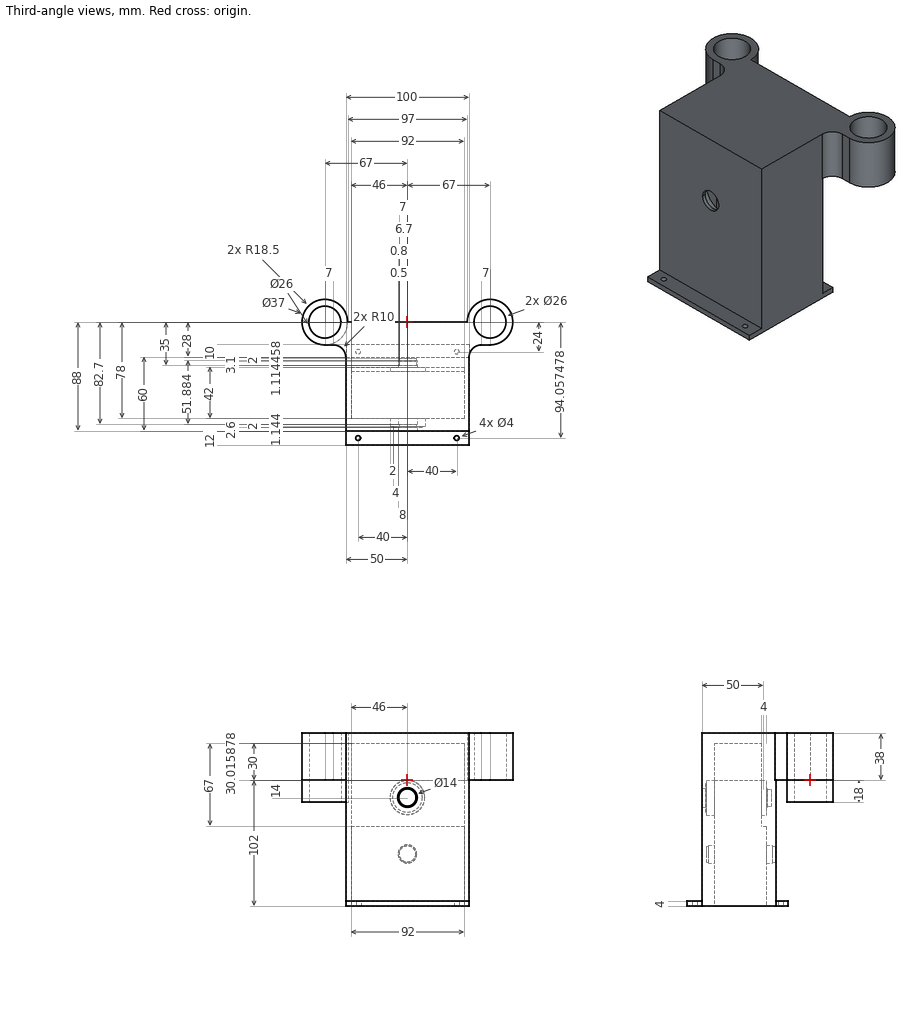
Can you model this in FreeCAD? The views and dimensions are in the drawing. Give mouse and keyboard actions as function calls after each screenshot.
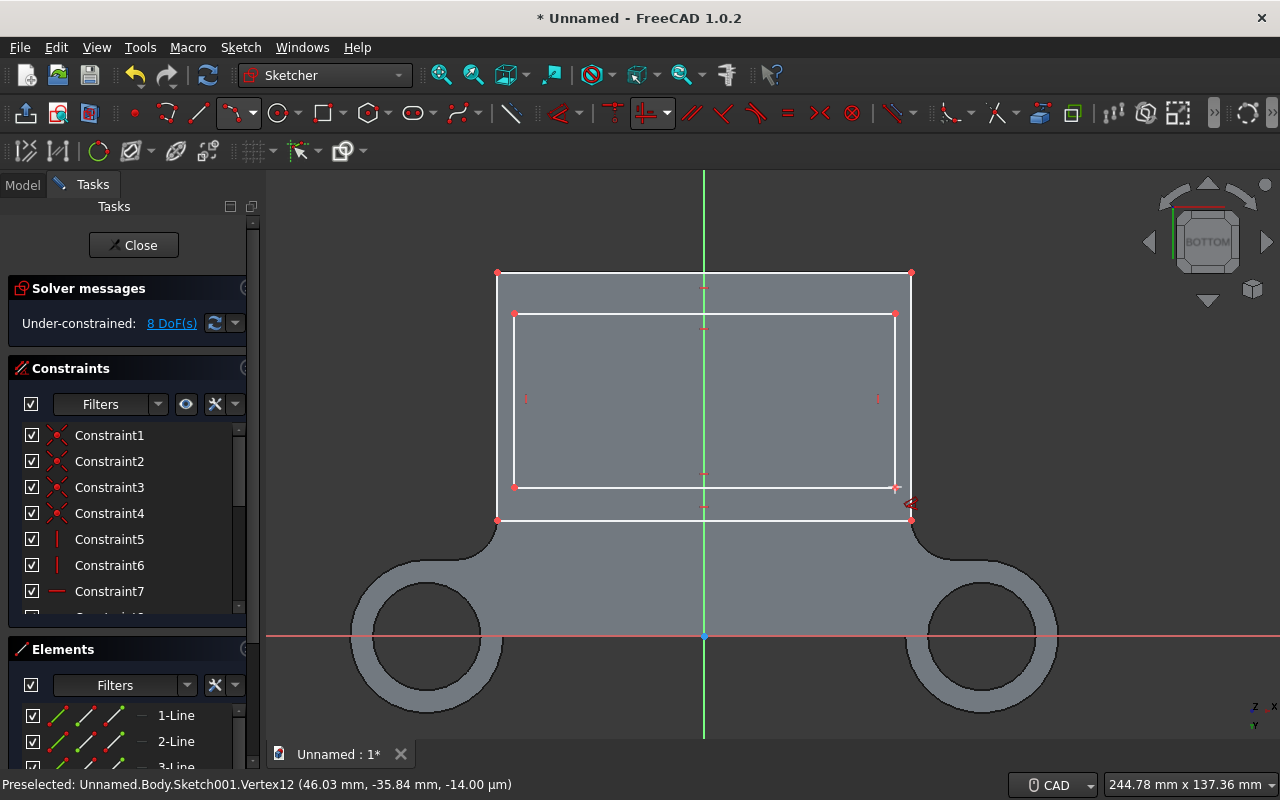
click(497, 347)
click(463, 397)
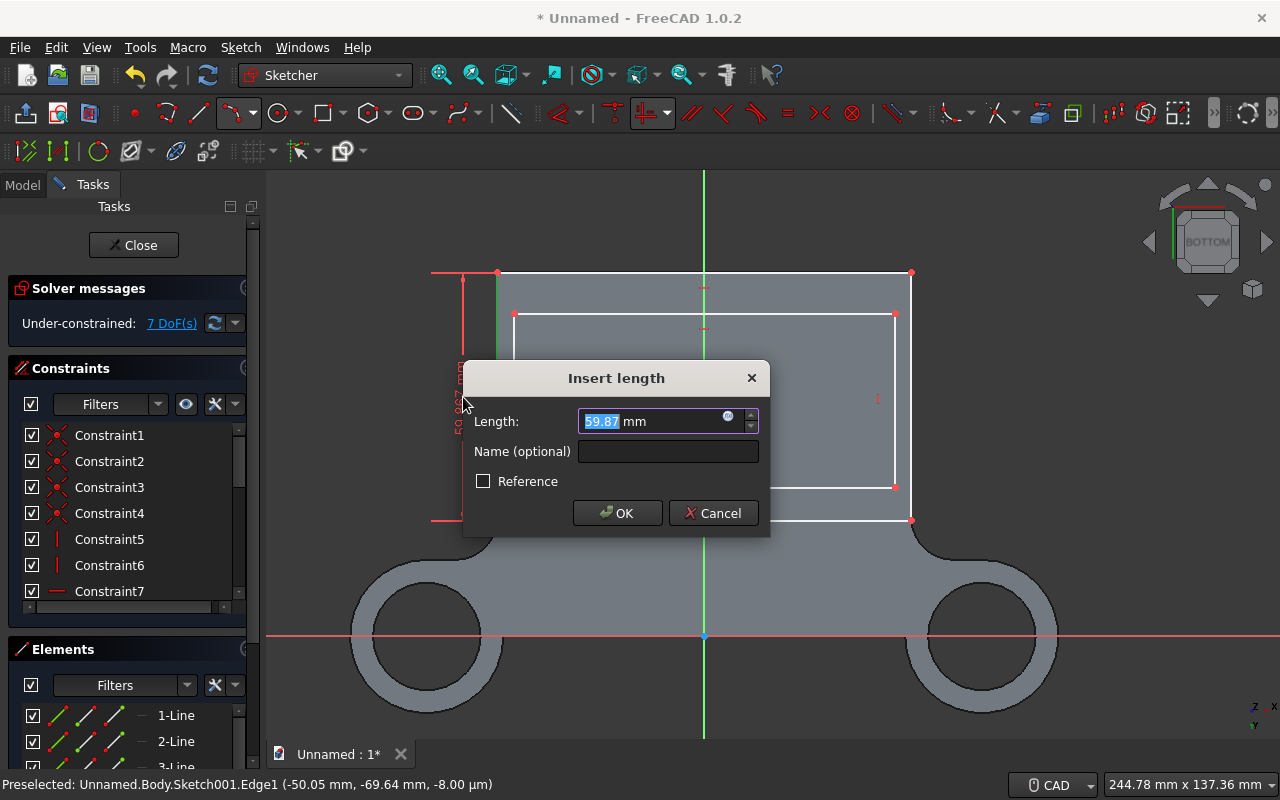
text(60)
key(Return)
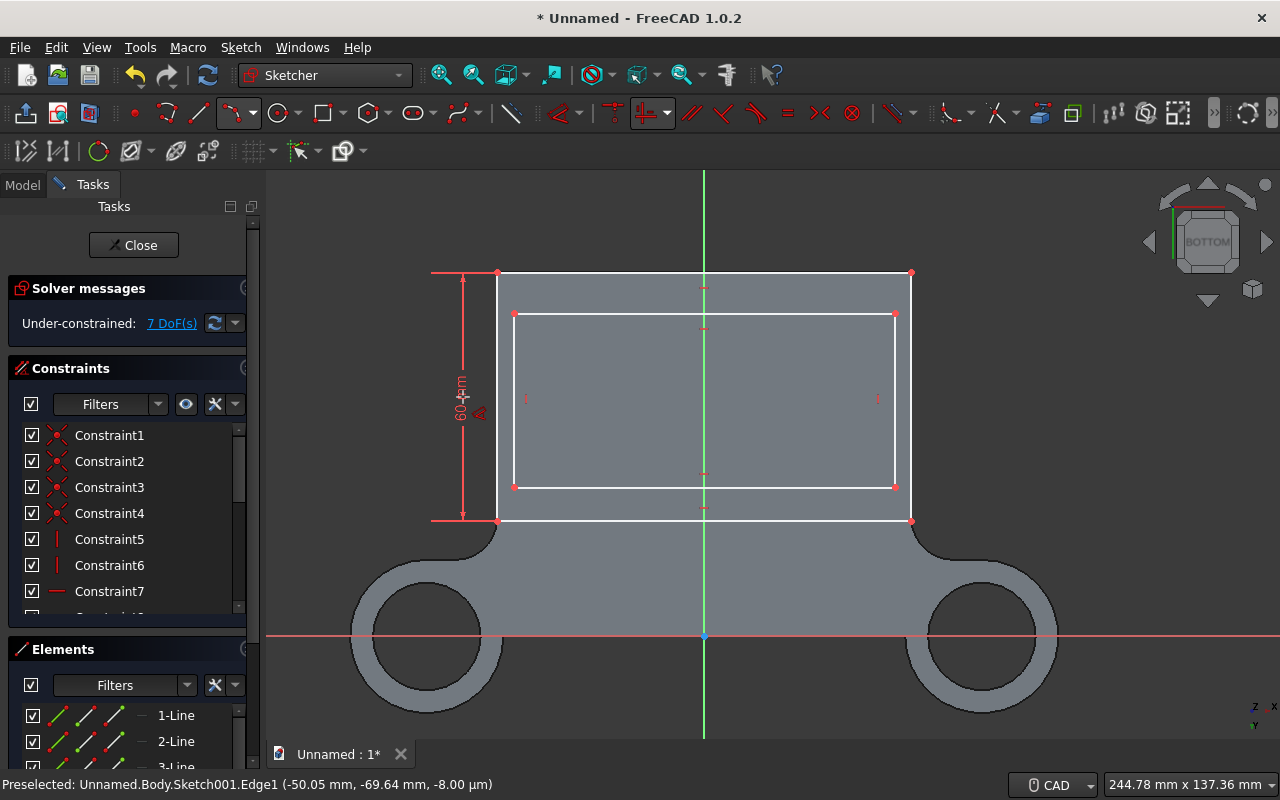
click(514, 366)
click(480, 361)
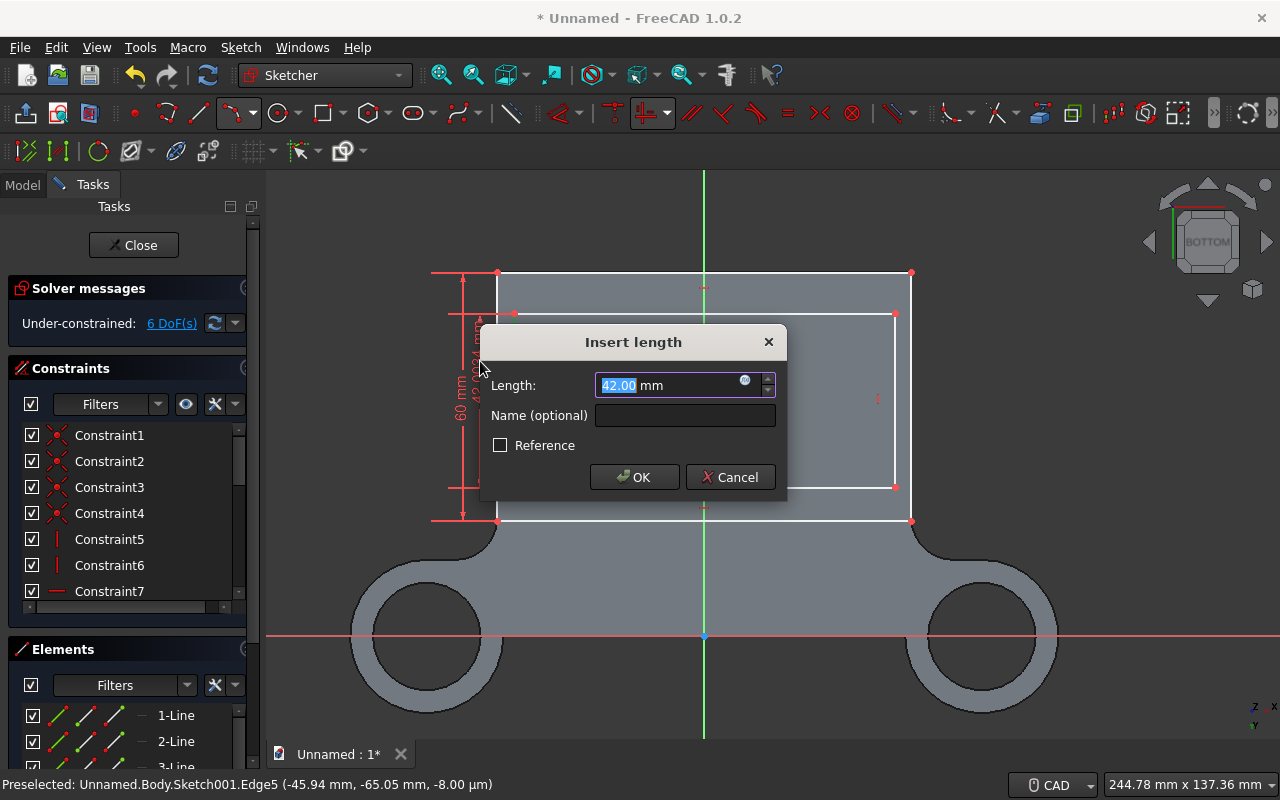
text(42)
key(Return)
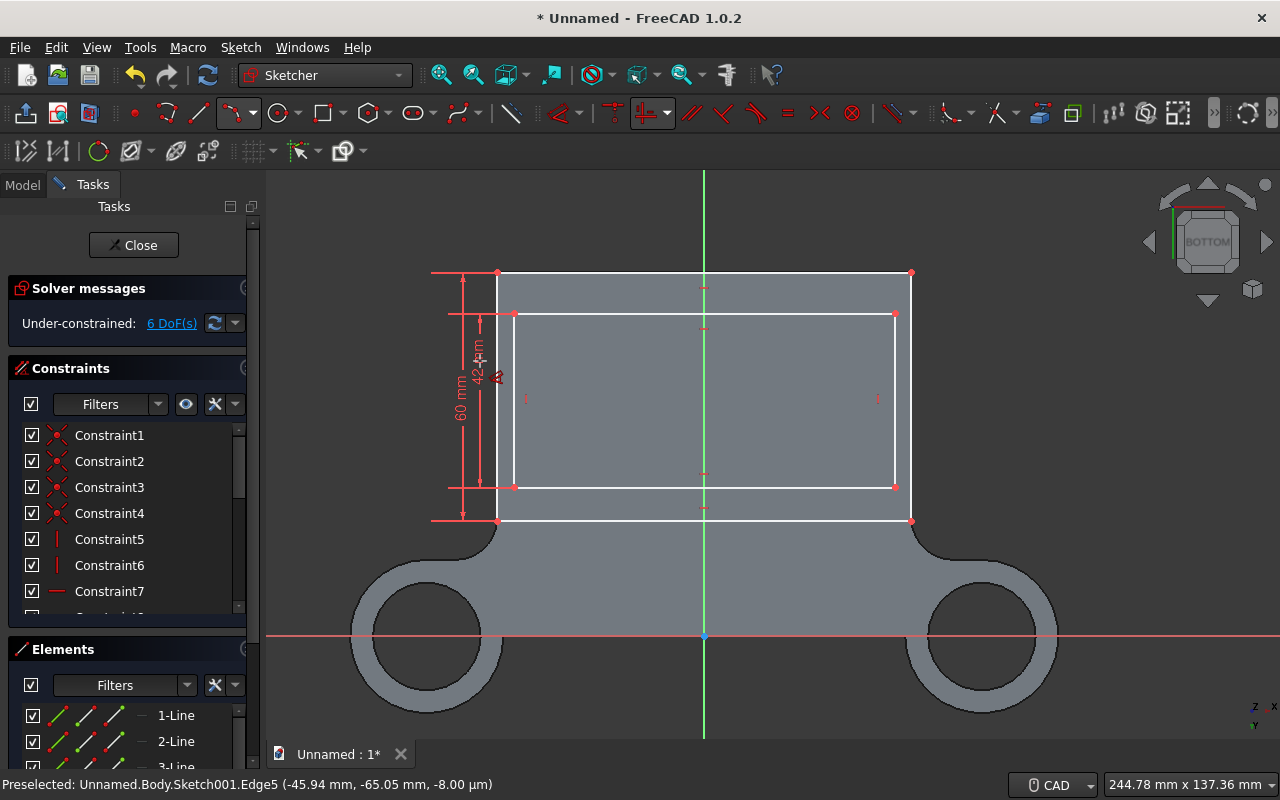
click(628, 488)
click(617, 454)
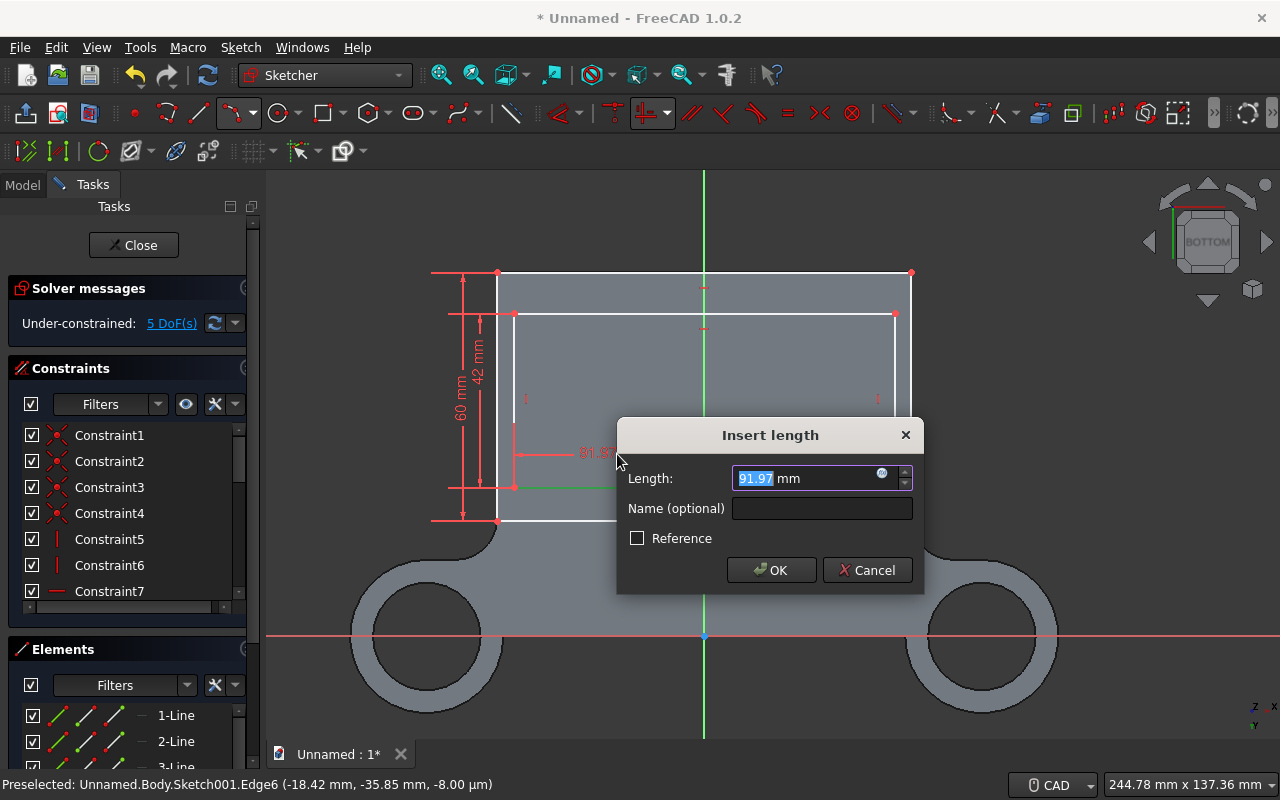
text(92)
key(Return)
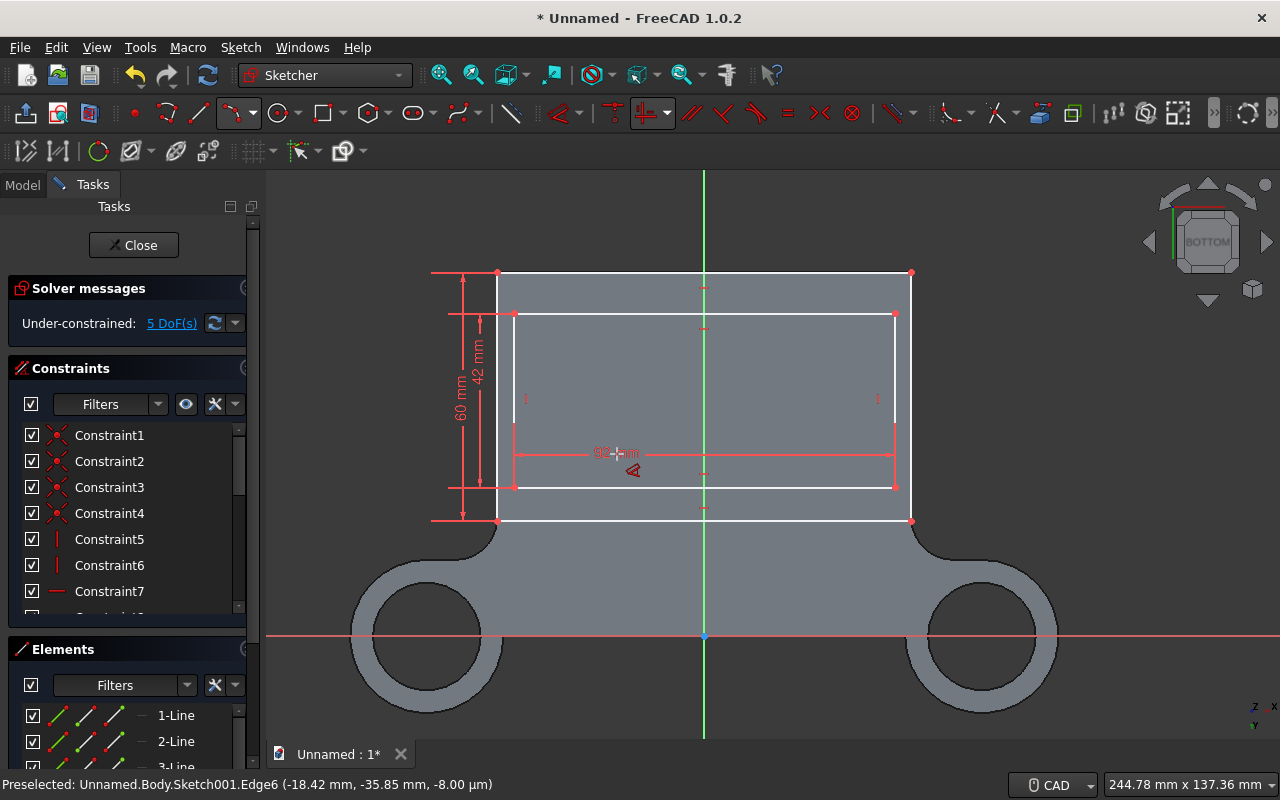
click(621, 521)
click(609, 555)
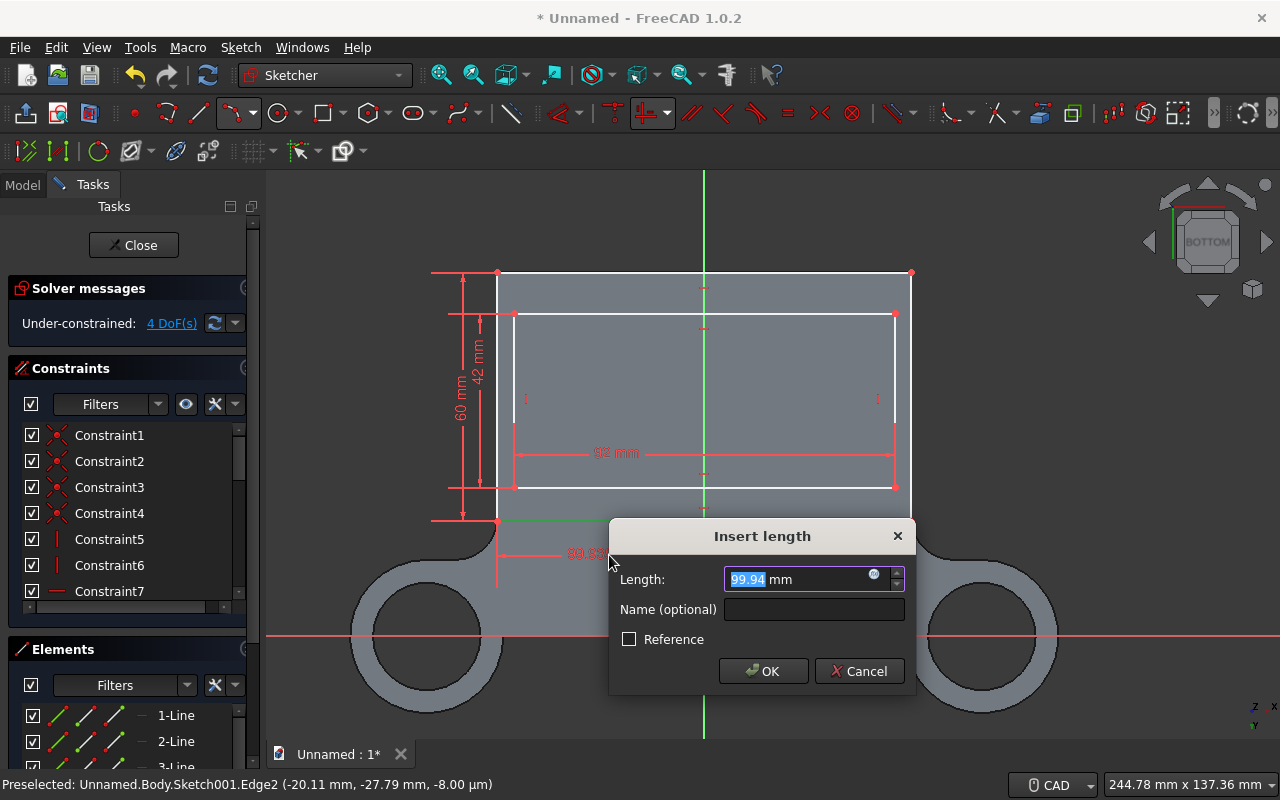
text(100)
key(Return)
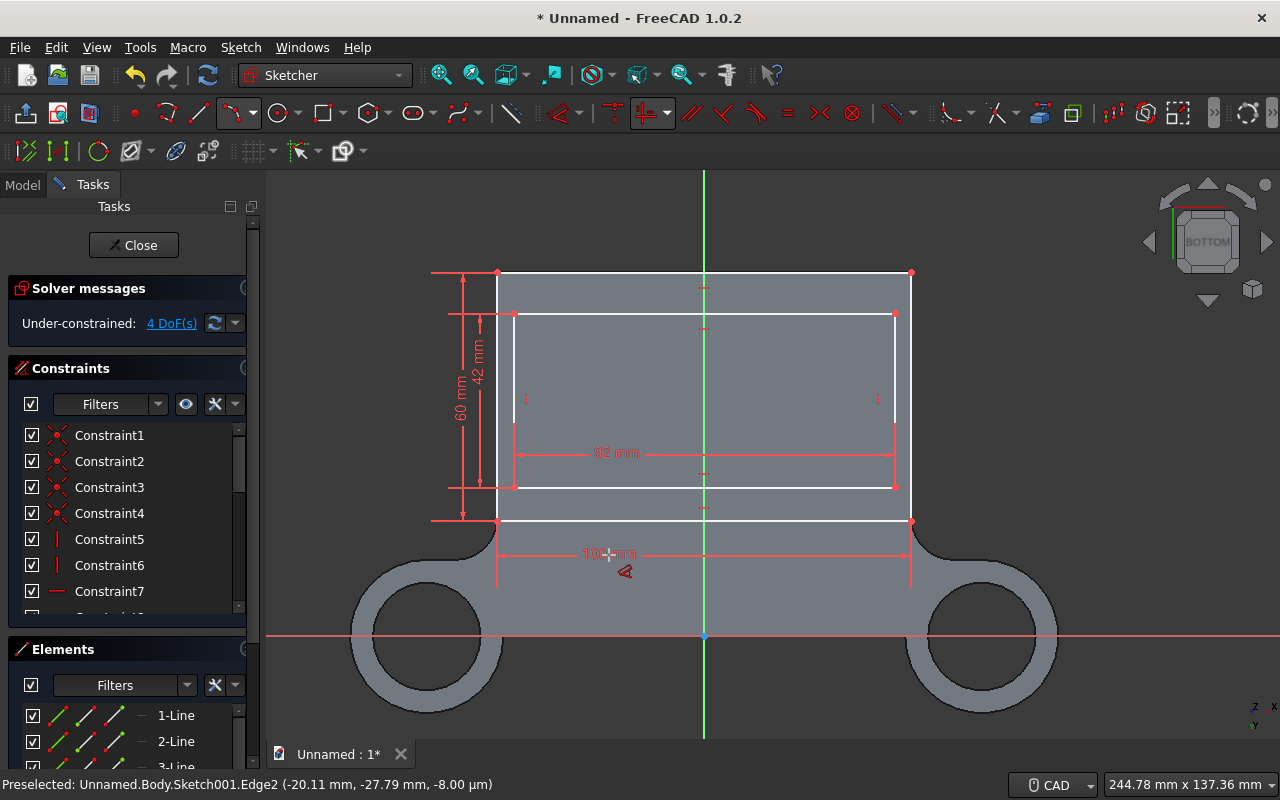
click(497, 273)
click(601, 670)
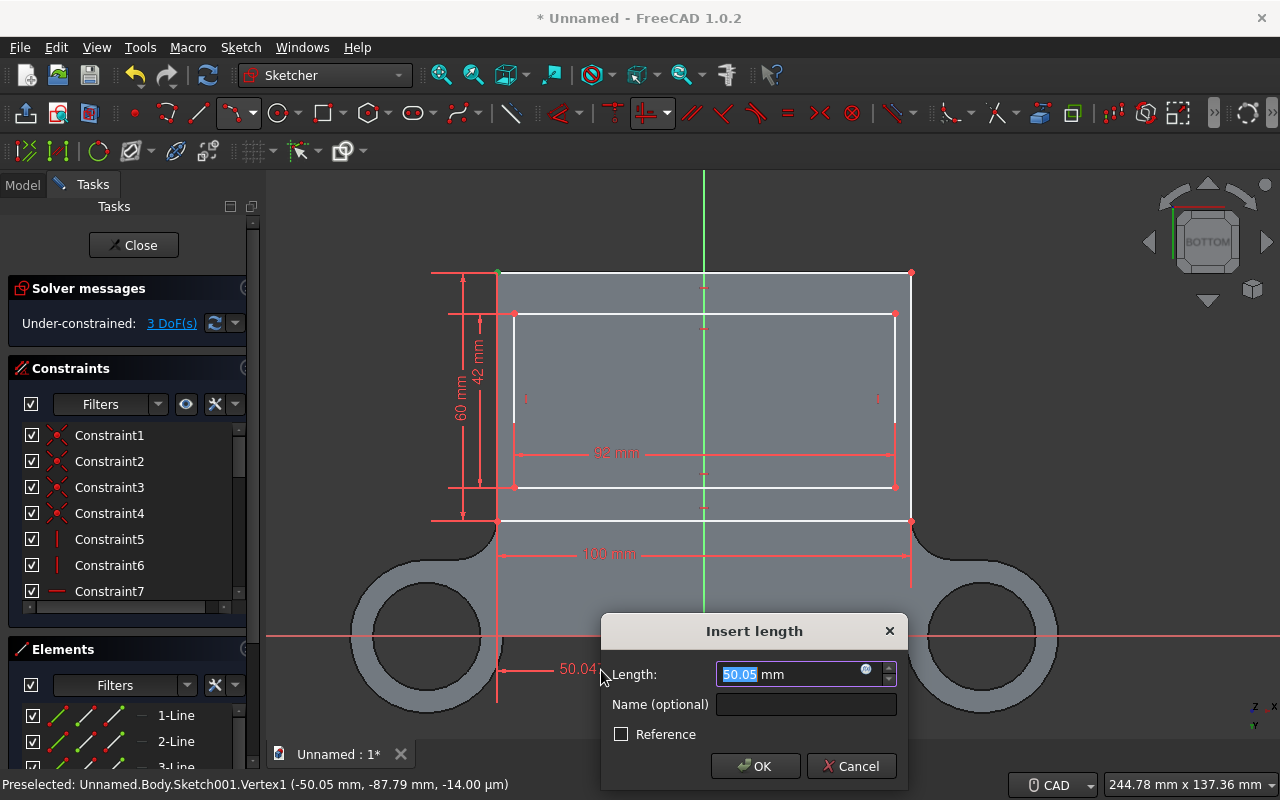
text(50)
key(Return)